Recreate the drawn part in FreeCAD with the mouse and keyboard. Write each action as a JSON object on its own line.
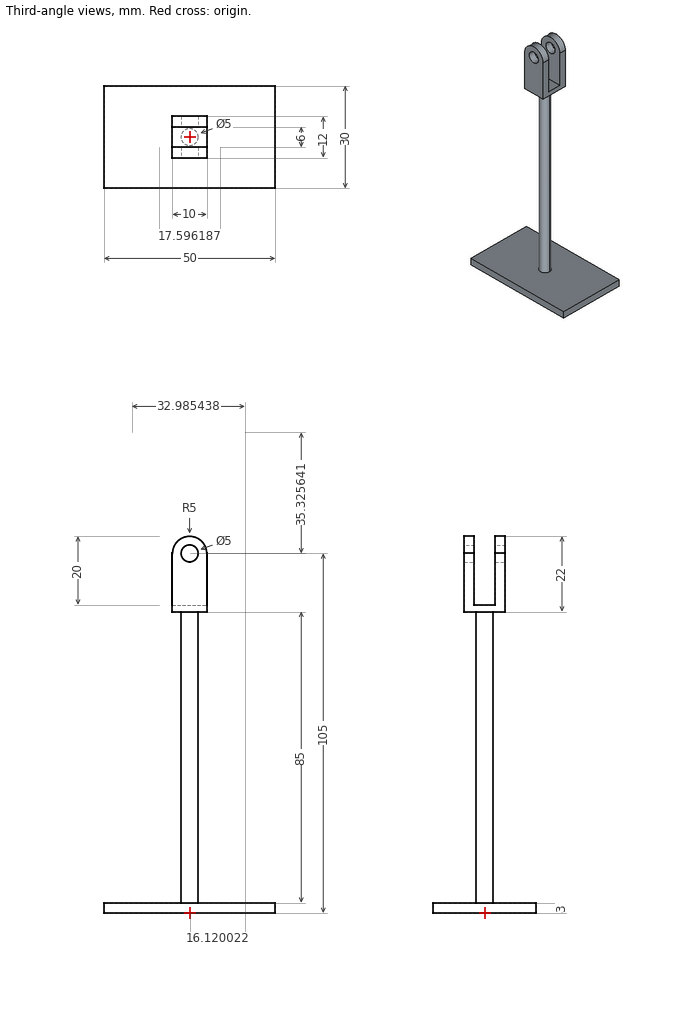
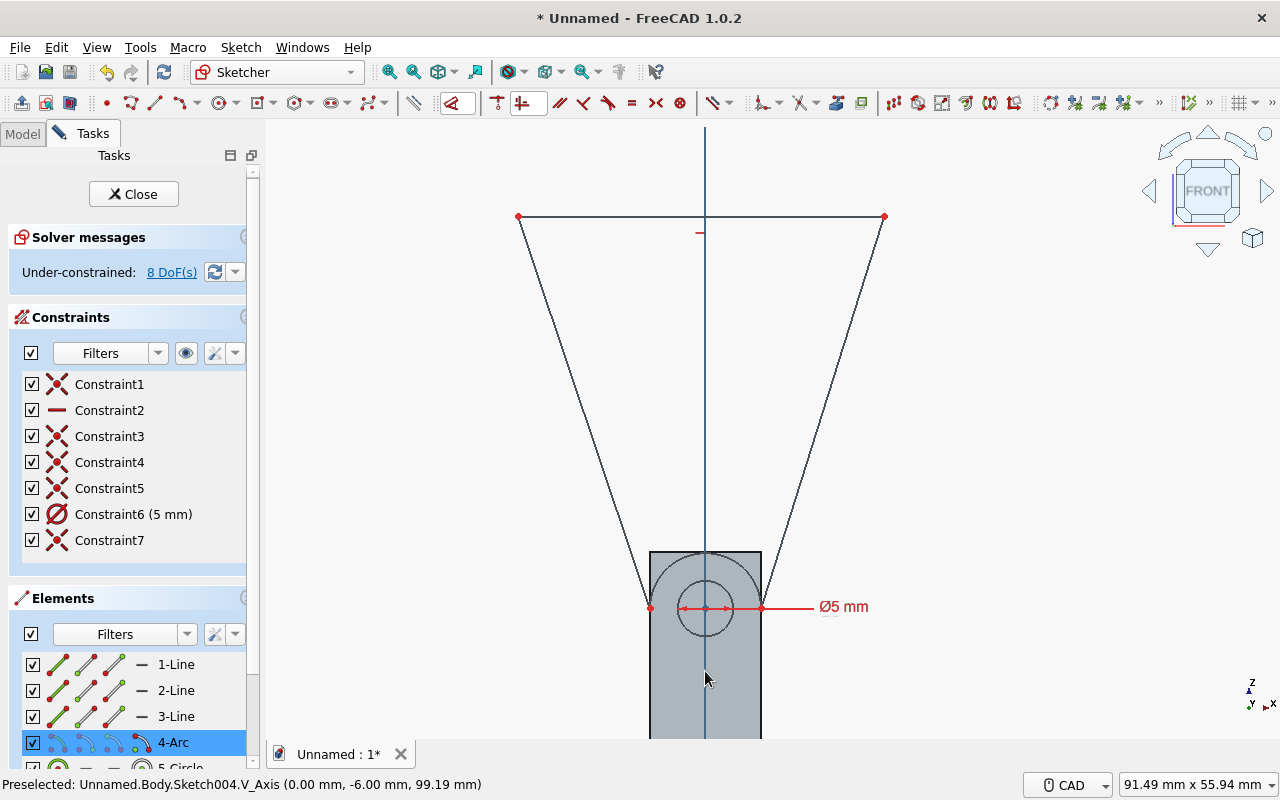
{"action": "left_click", "coordinate": [498, 104]}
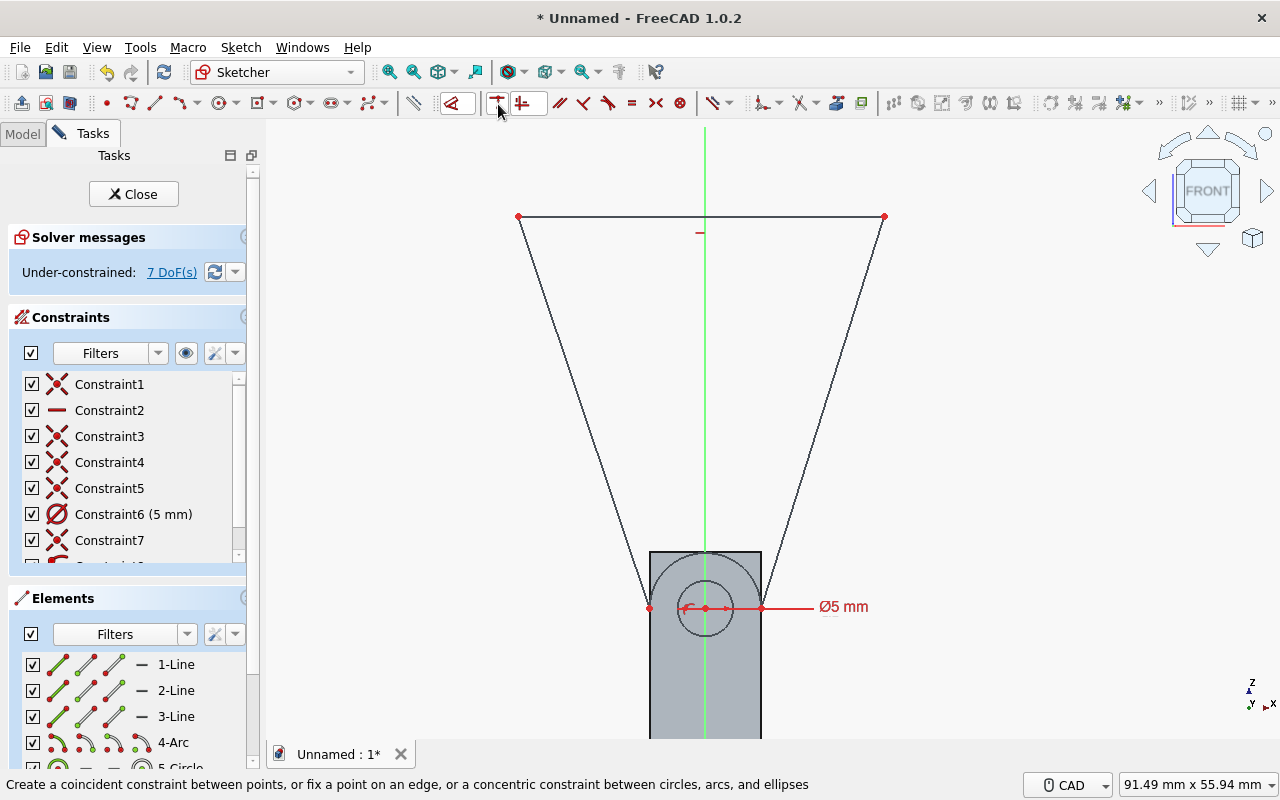
{"action": "left_click", "coordinate": [452, 104]}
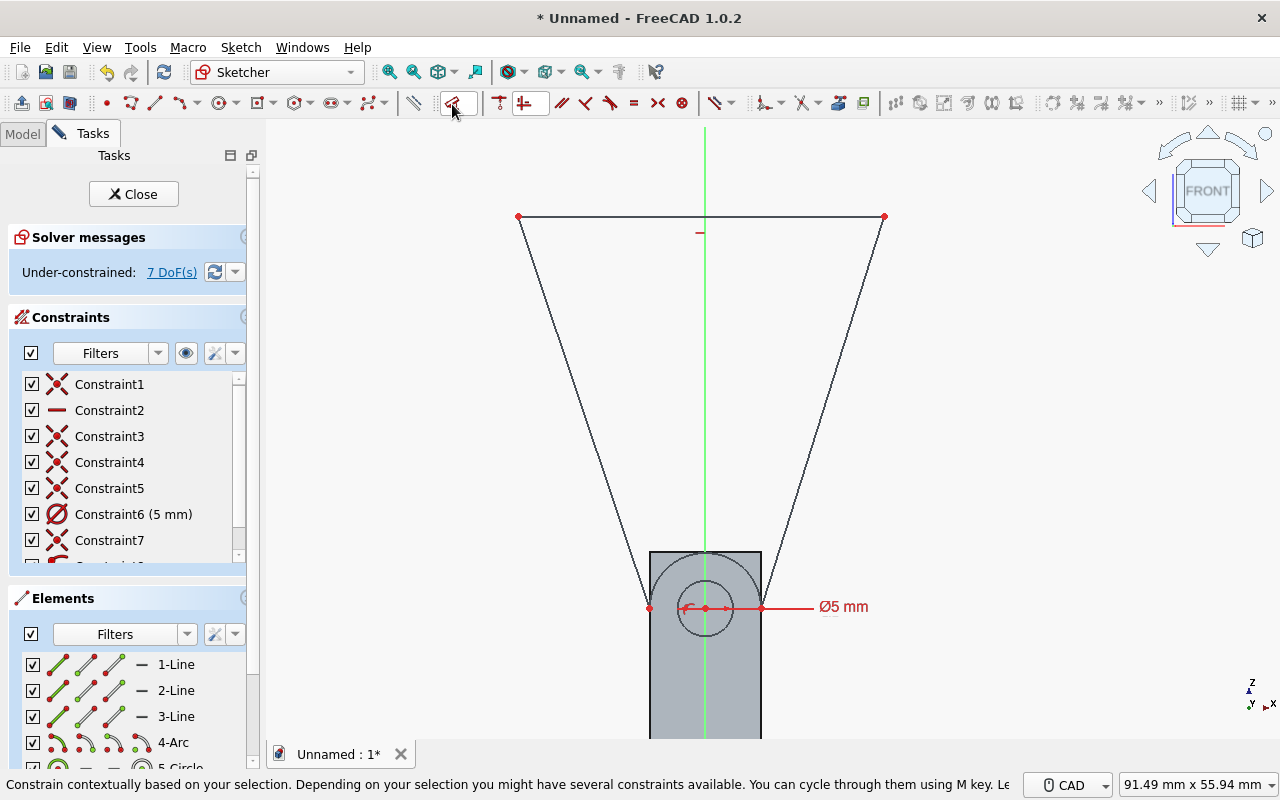
{"action": "left_click", "coordinate": [738, 564]}
{"action": "left_click", "coordinate": [757, 538]}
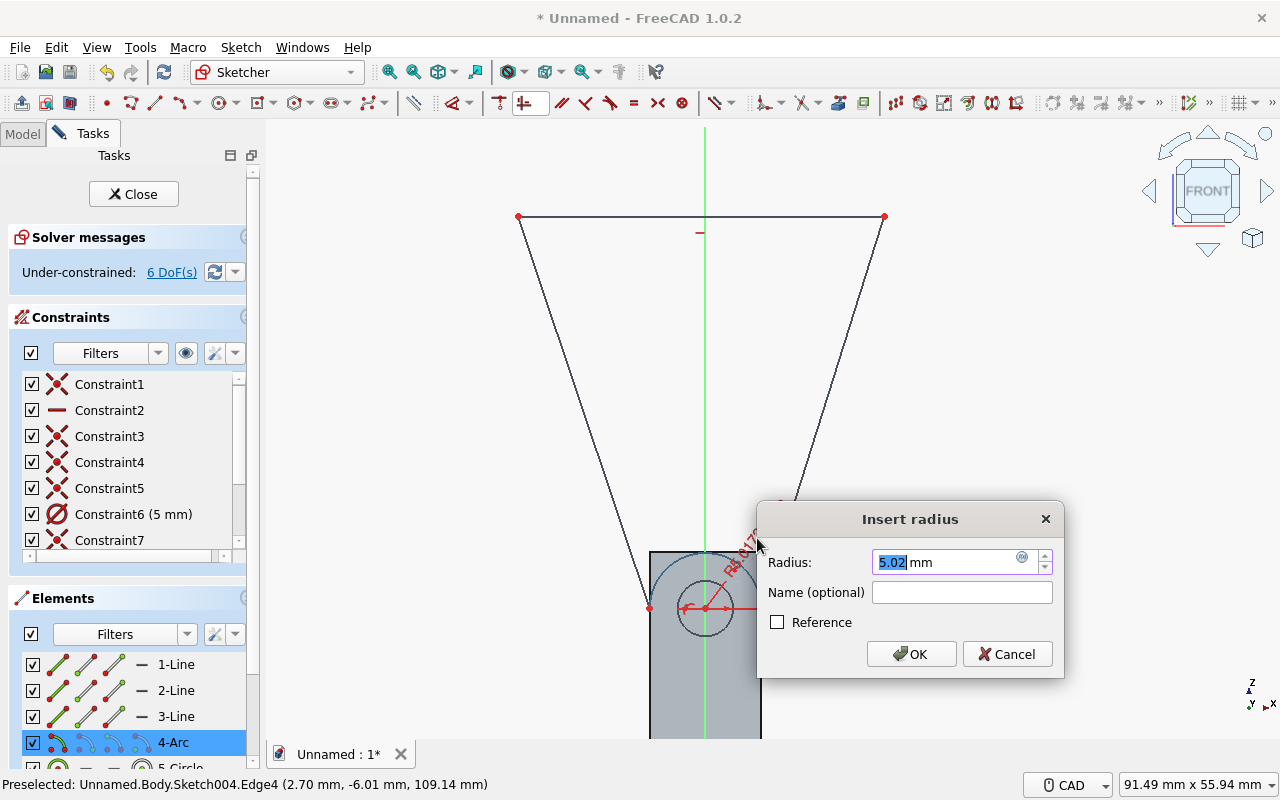
{"action": "type", "text": "5"}
{"action": "key", "text": "Return"}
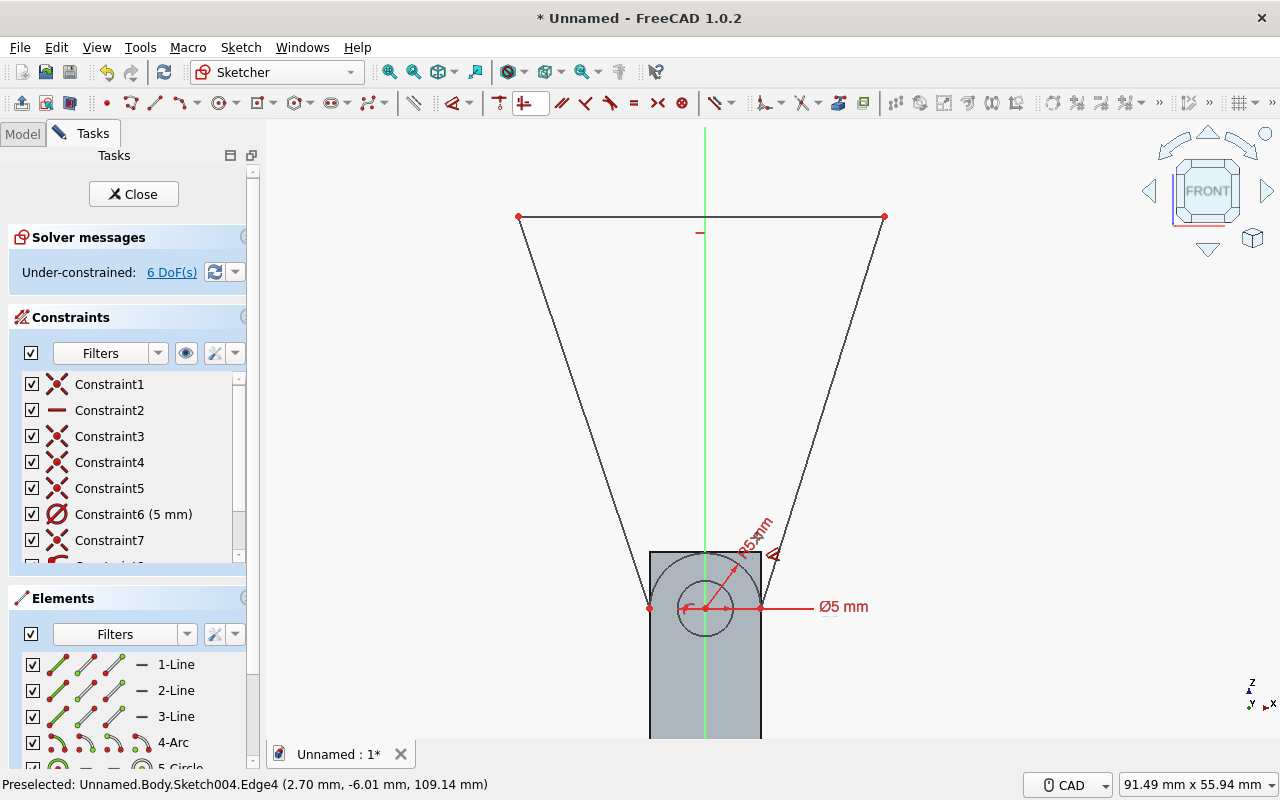
{"action": "left_click", "coordinate": [705, 609]}
{"action": "left_click", "coordinate": [739, 660]}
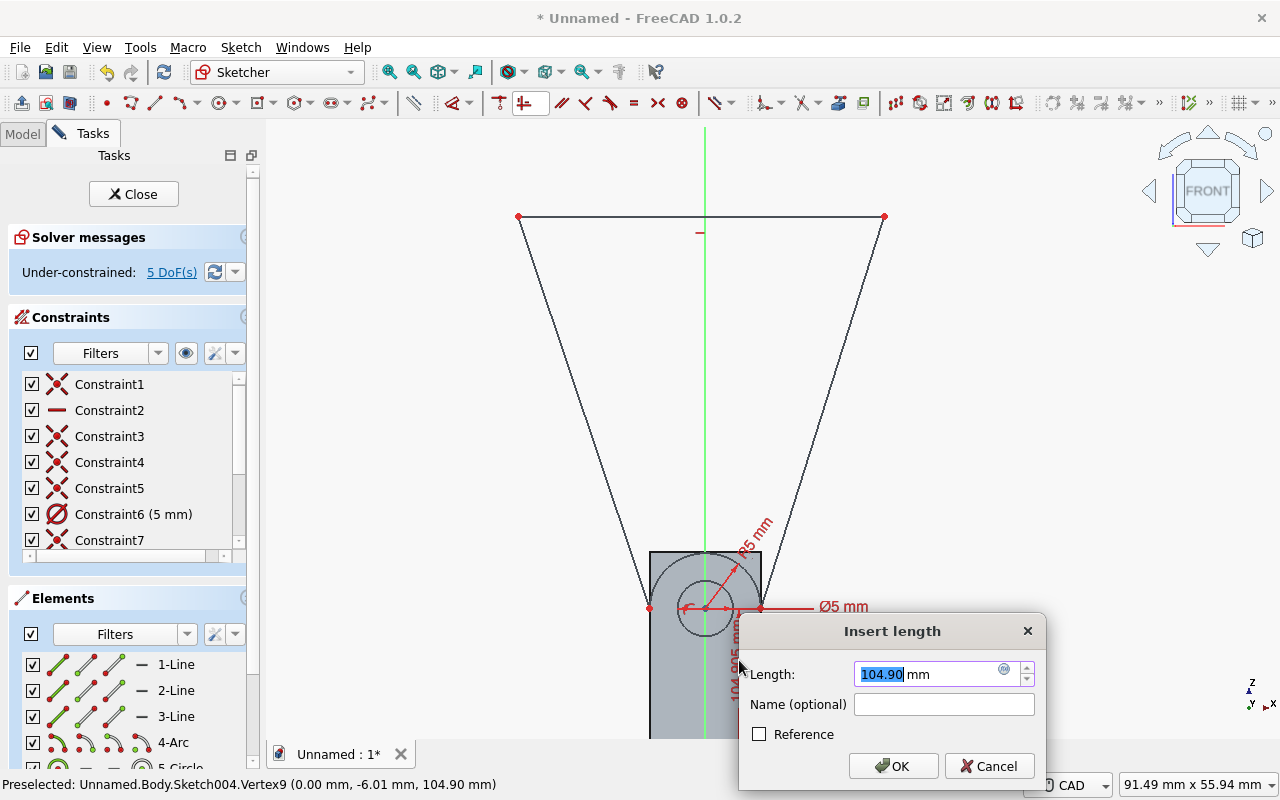
{"action": "type", "text": "105"}
{"action": "key", "text": "Return"}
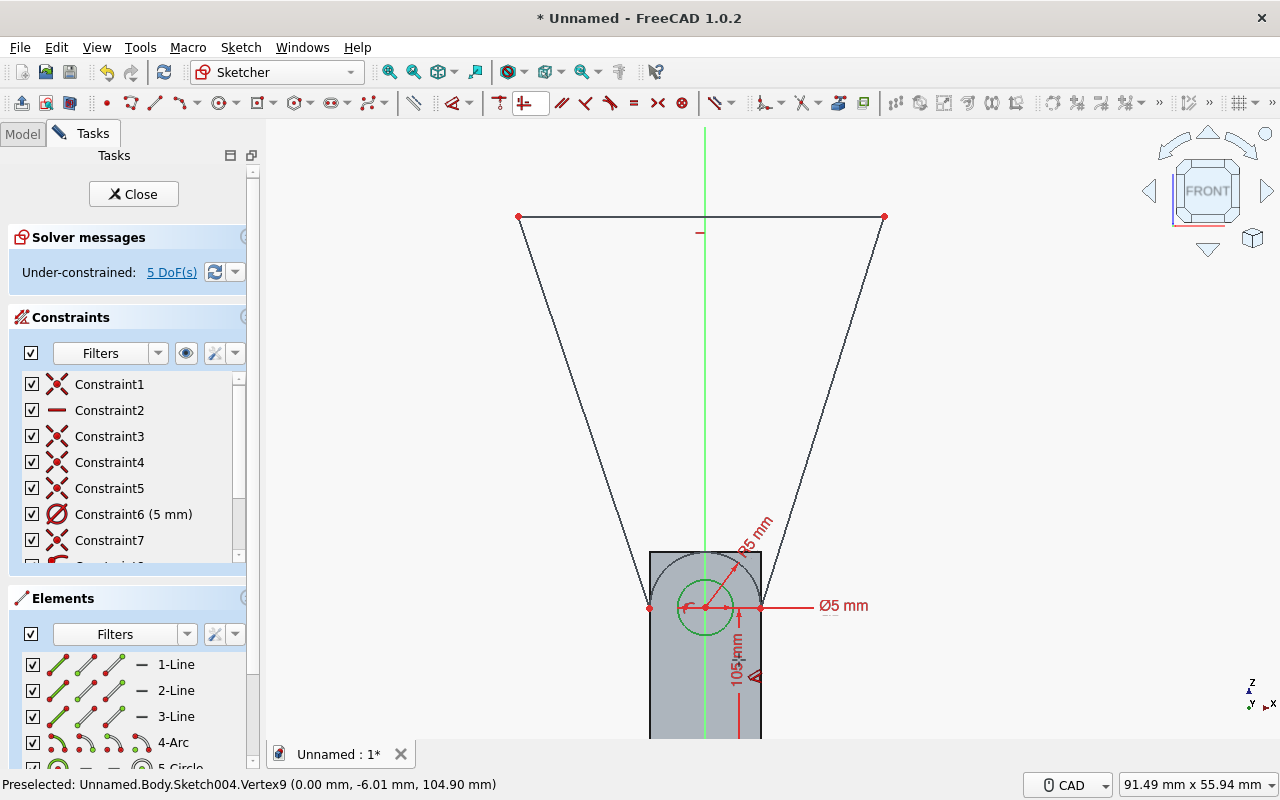
{"action": "left_click", "coordinate": [761, 609]}
{"action": "left_click", "coordinate": [795, 637]}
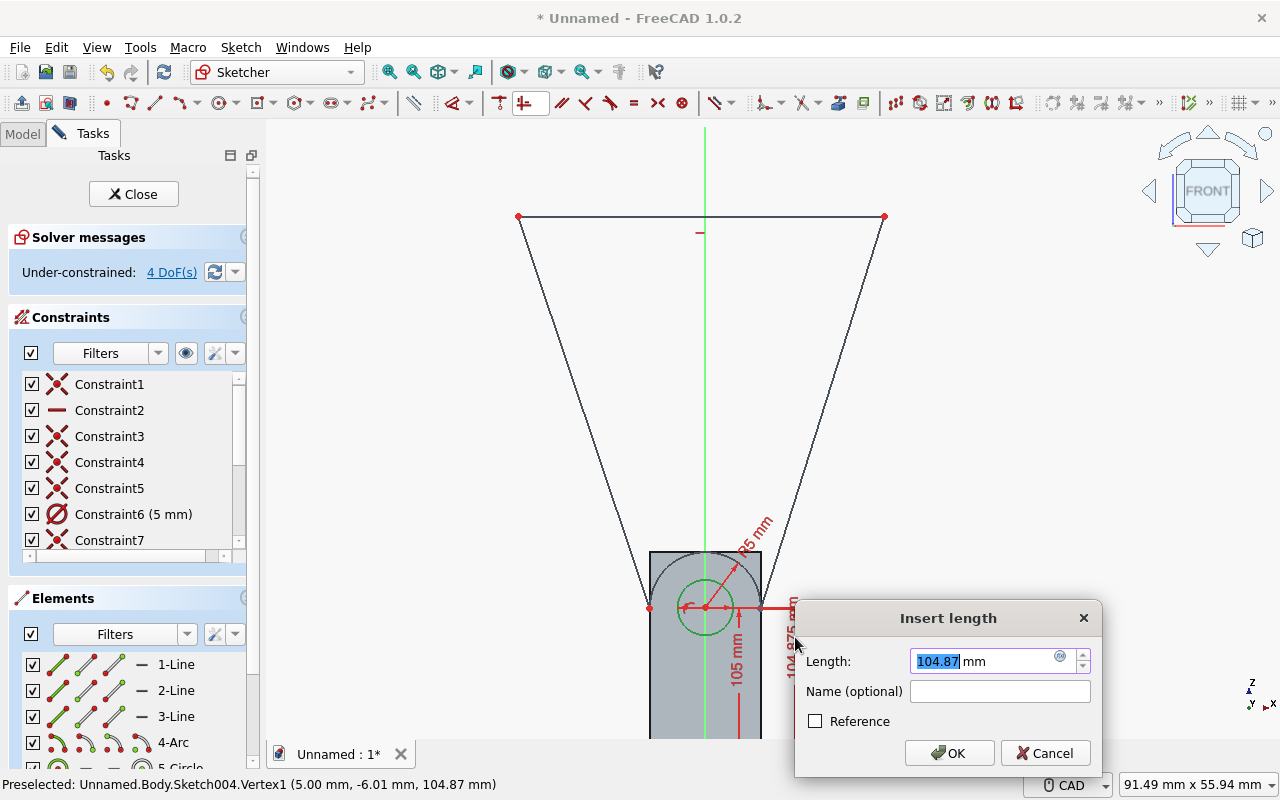
{"action": "type", "text": "105"}
{"action": "key", "text": "Return"}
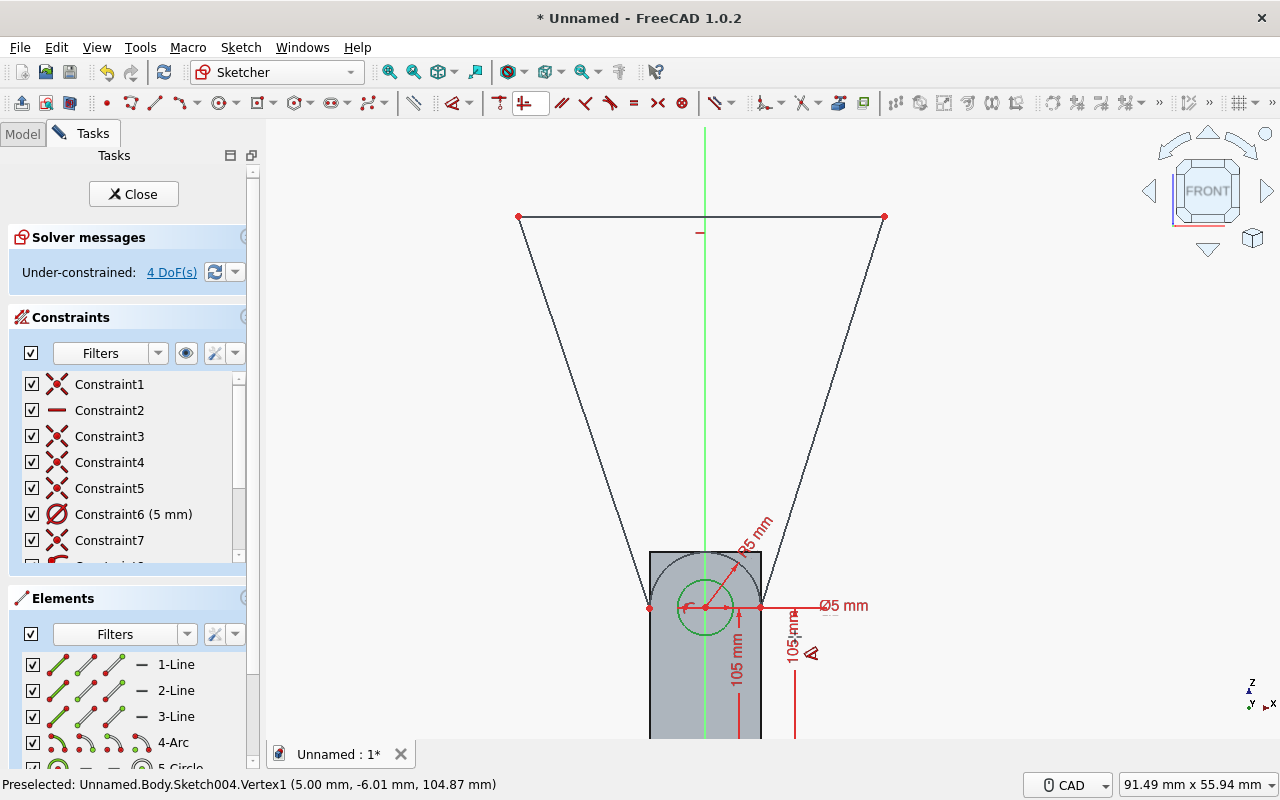
{"action": "left_click", "coordinate": [650, 609]}
{"action": "left_click", "coordinate": [616, 660]}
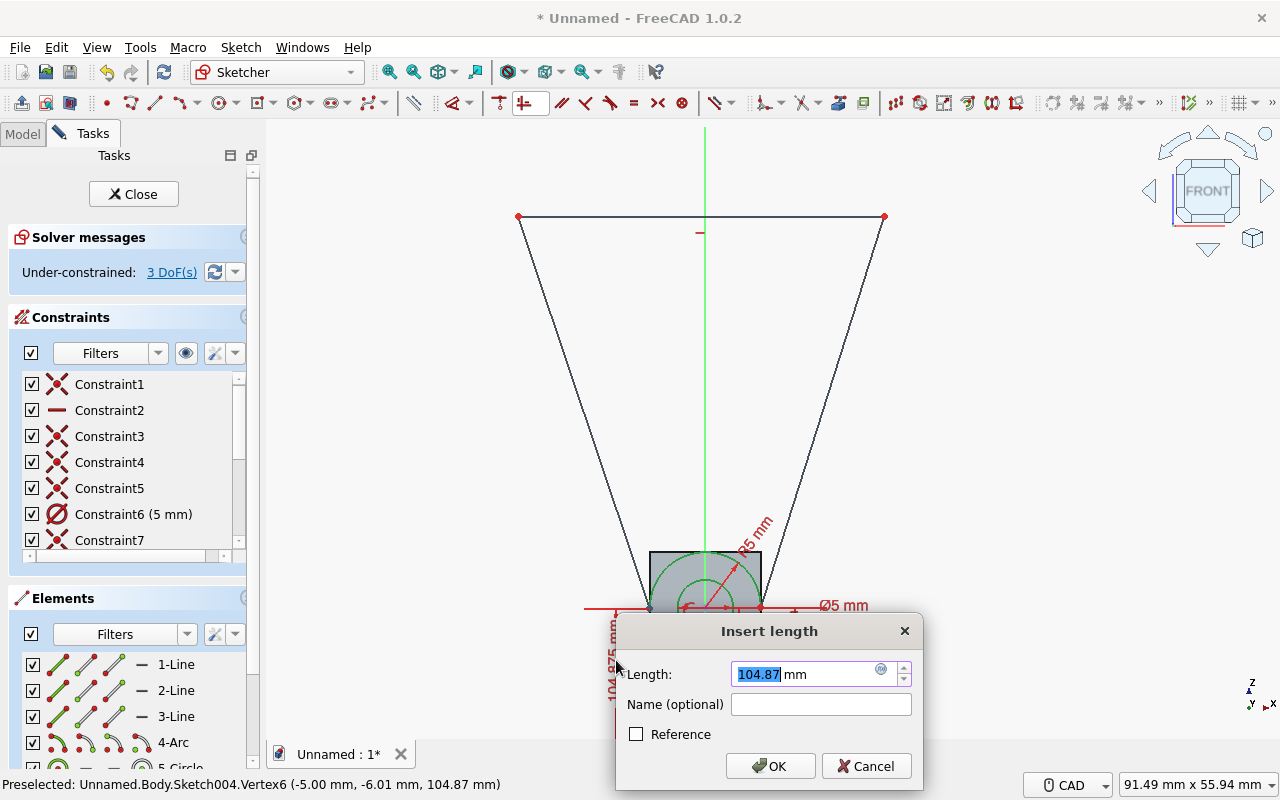
{"action": "type", "text": "105"}
{"action": "key", "text": "Return"}